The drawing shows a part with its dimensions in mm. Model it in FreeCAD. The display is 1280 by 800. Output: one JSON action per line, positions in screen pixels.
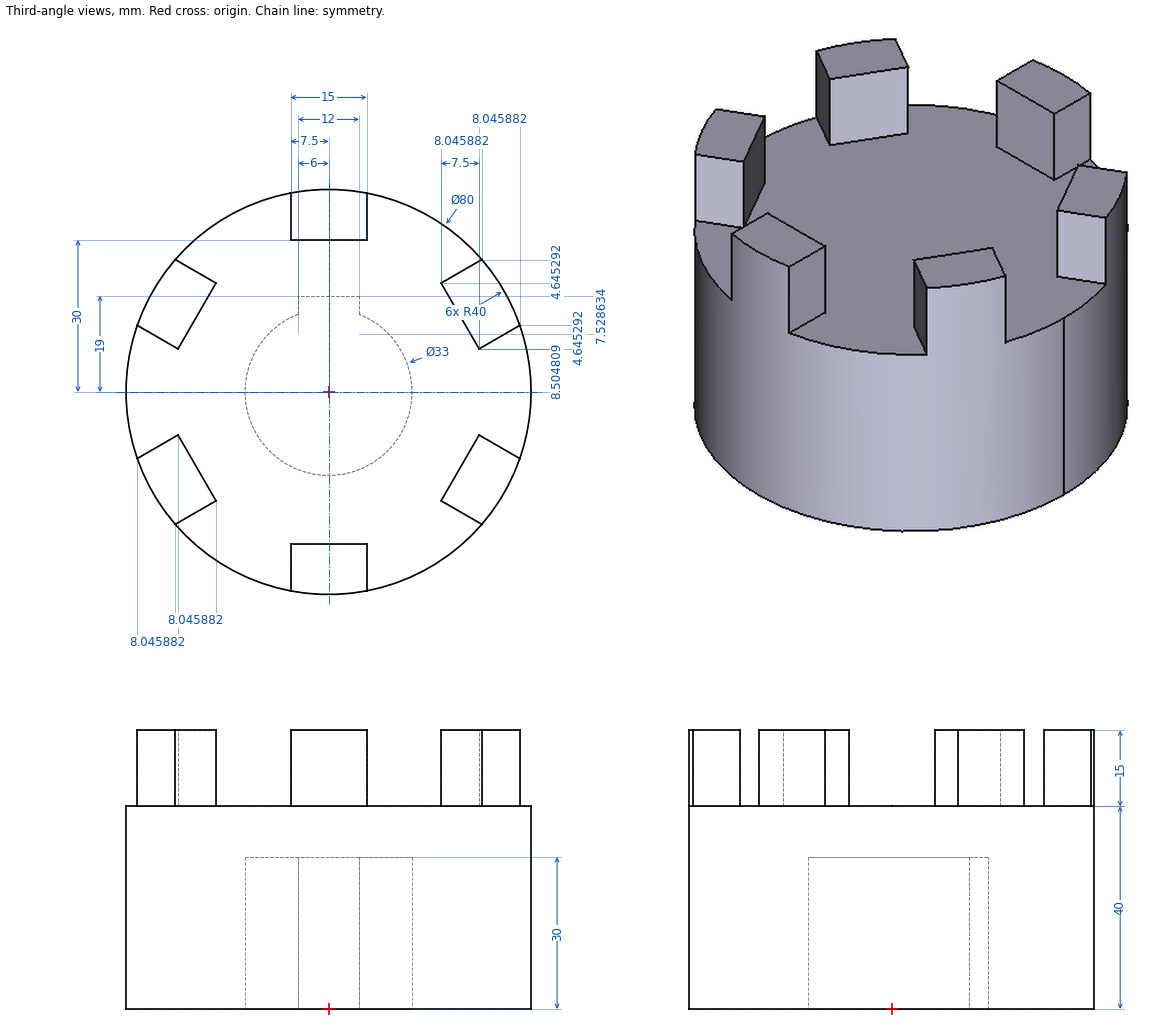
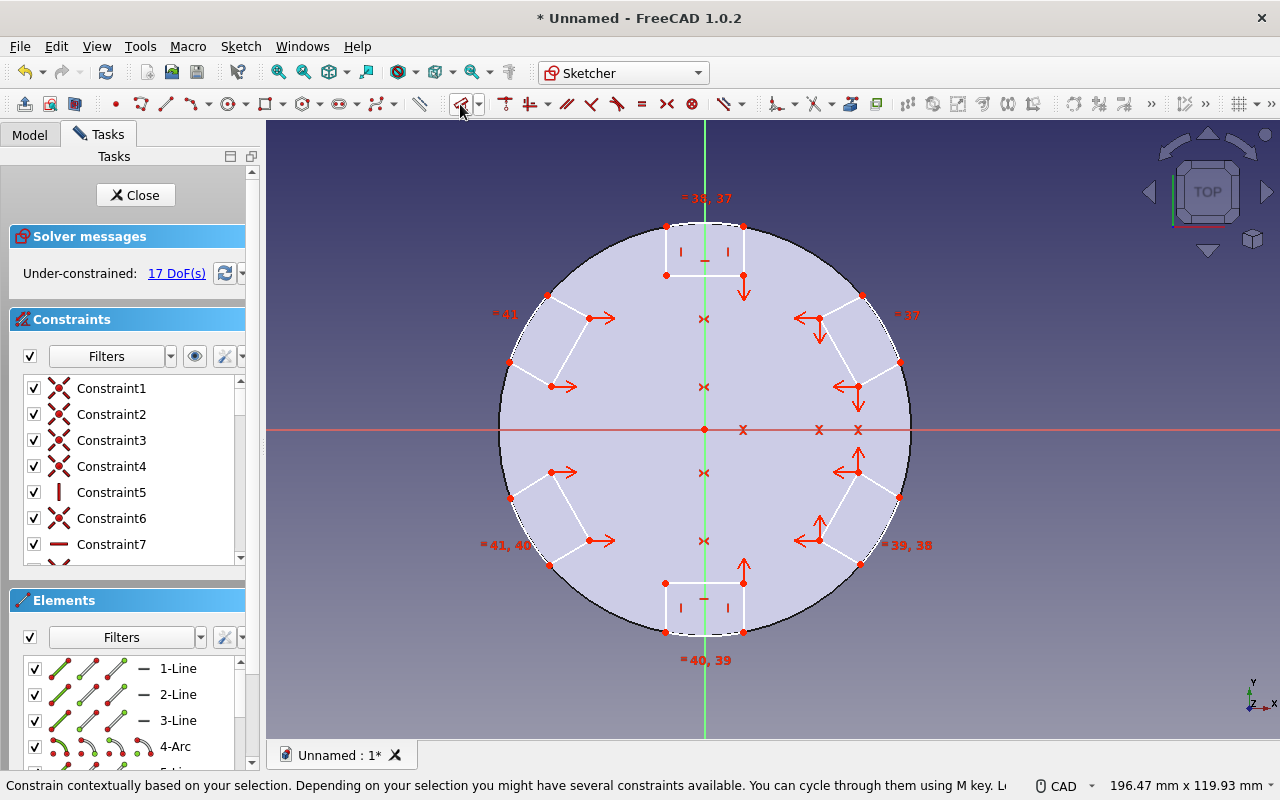
{"action": "left_click", "coordinate": [892, 341]}
{"action": "left_click", "coordinate": [921, 327]}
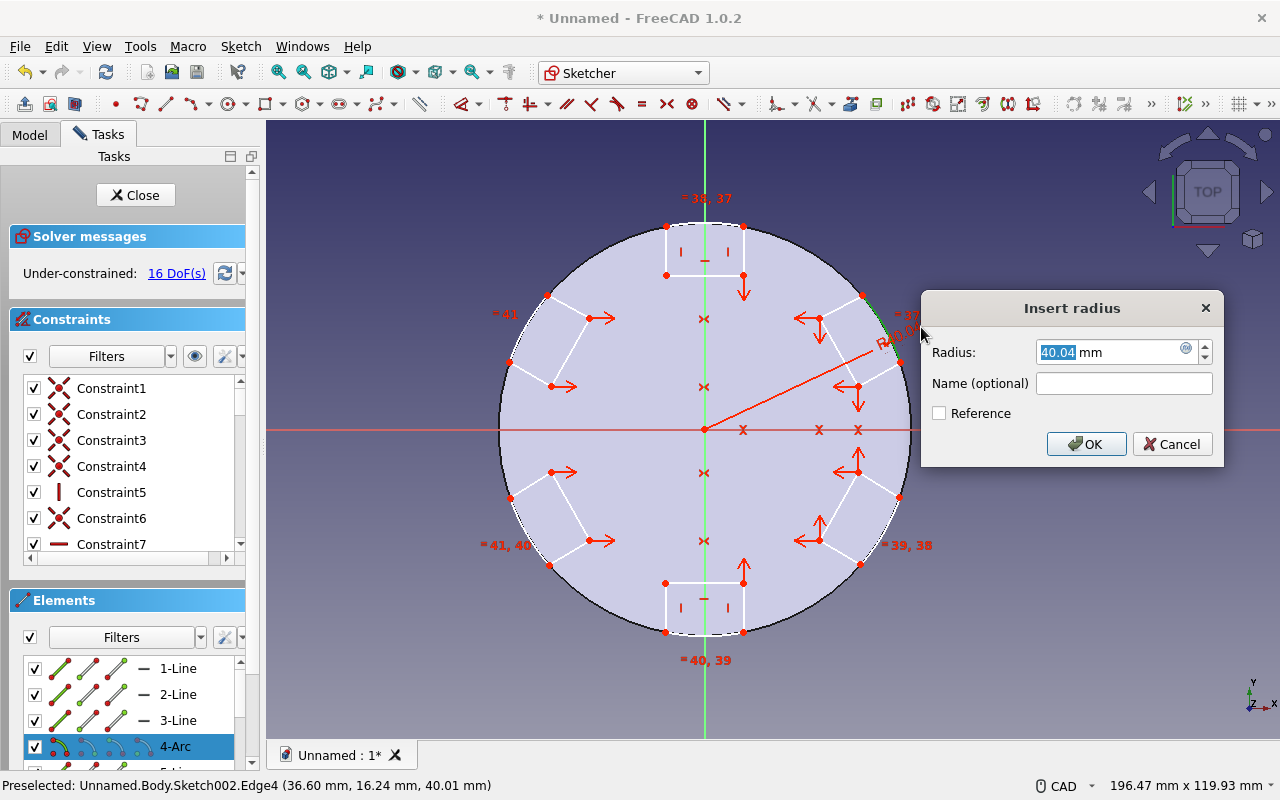
{"action": "type", "text": "40"}
{"action": "key", "text": "Return"}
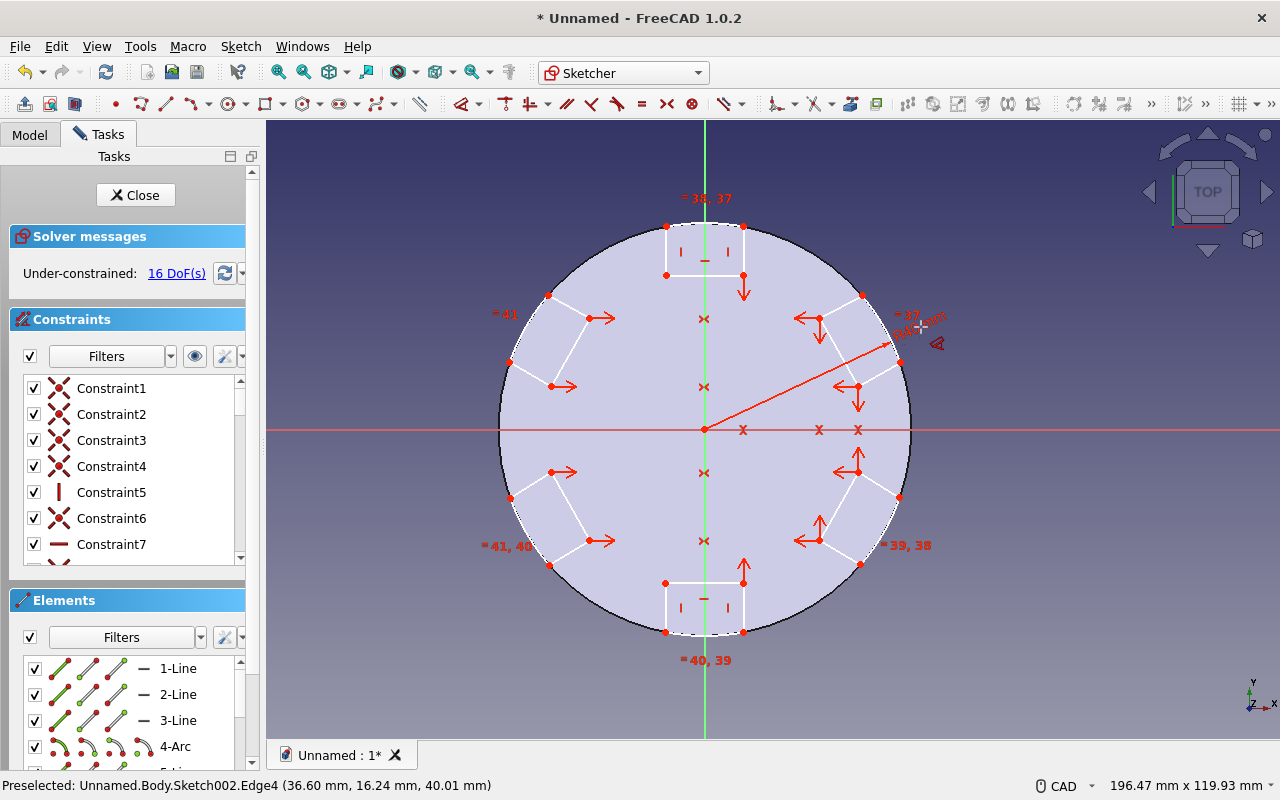
{"action": "left_click", "coordinate": [689, 276]}
{"action": "left_click", "coordinate": [687, 242]}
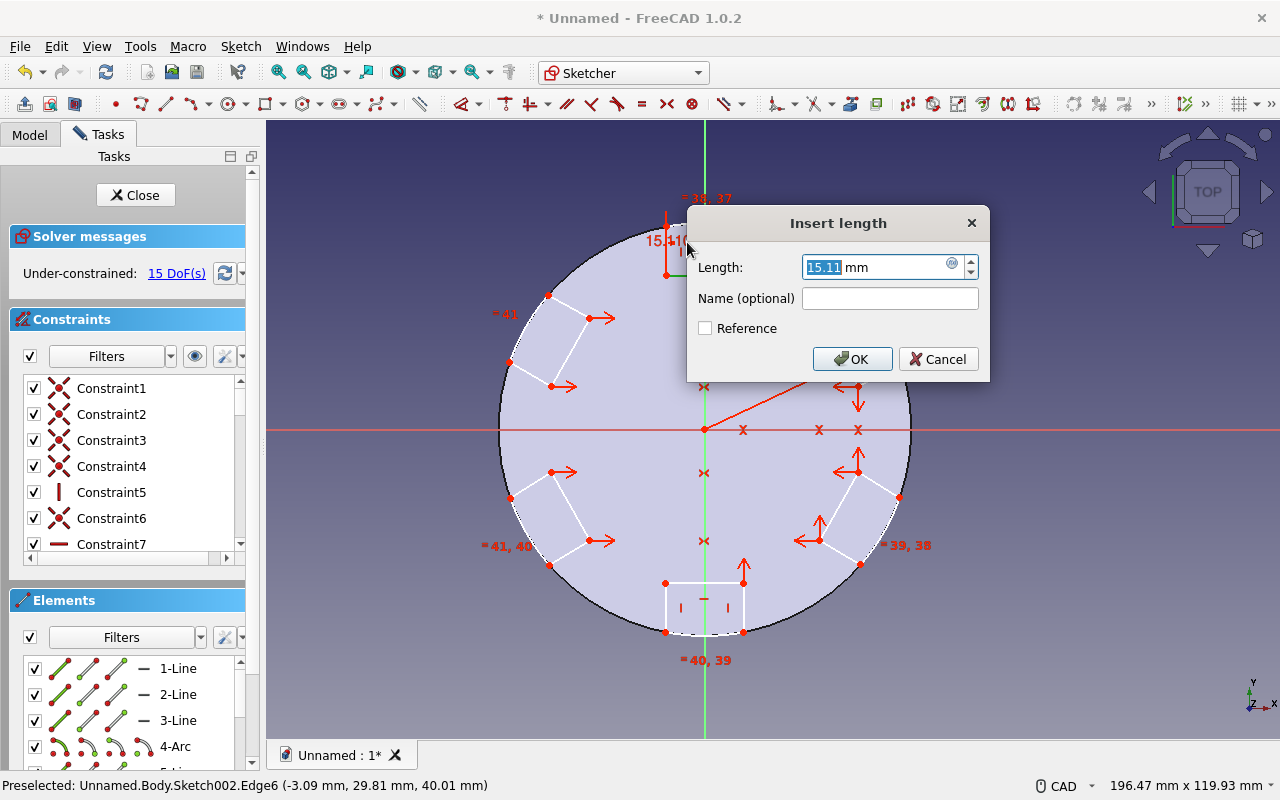
{"action": "type", "text": "15"}
{"action": "key", "text": "Return"}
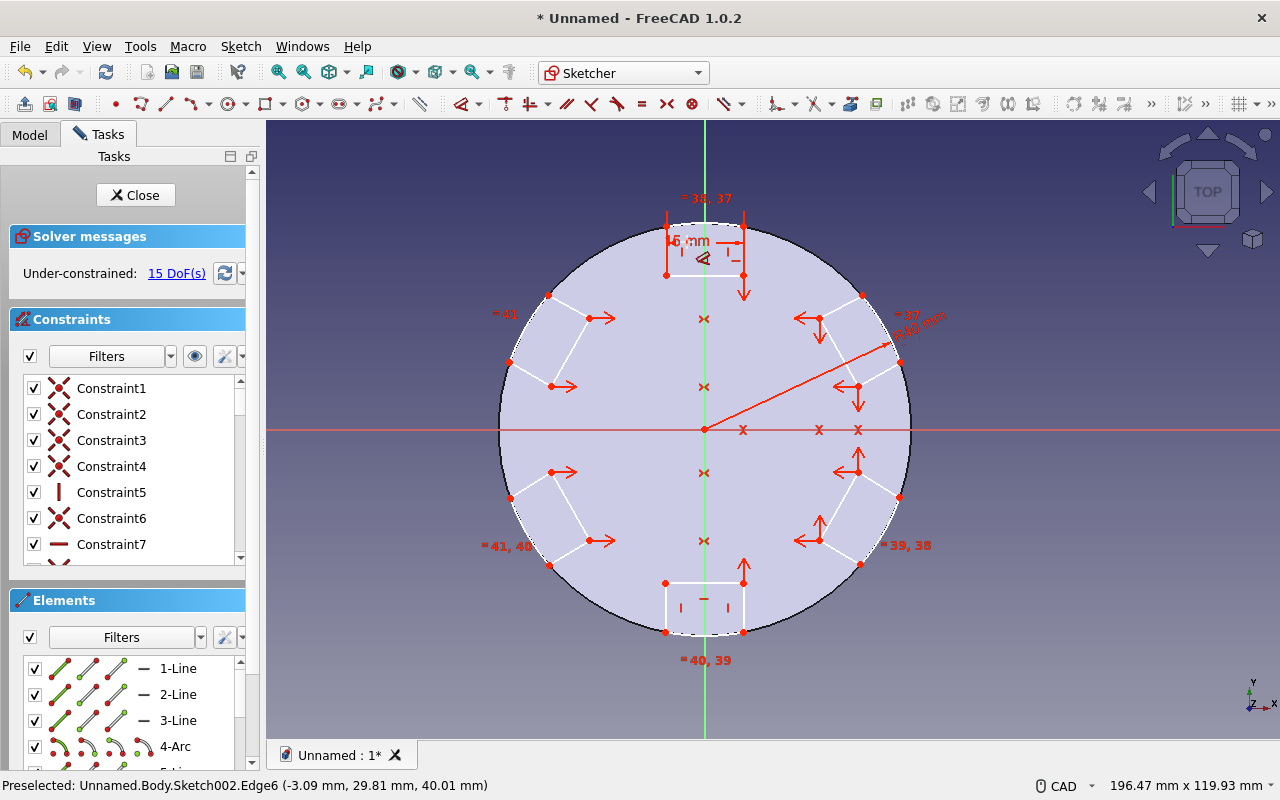
{"action": "left_click", "coordinate": [721, 583]}
{"action": "left_click", "coordinate": [687, 617]}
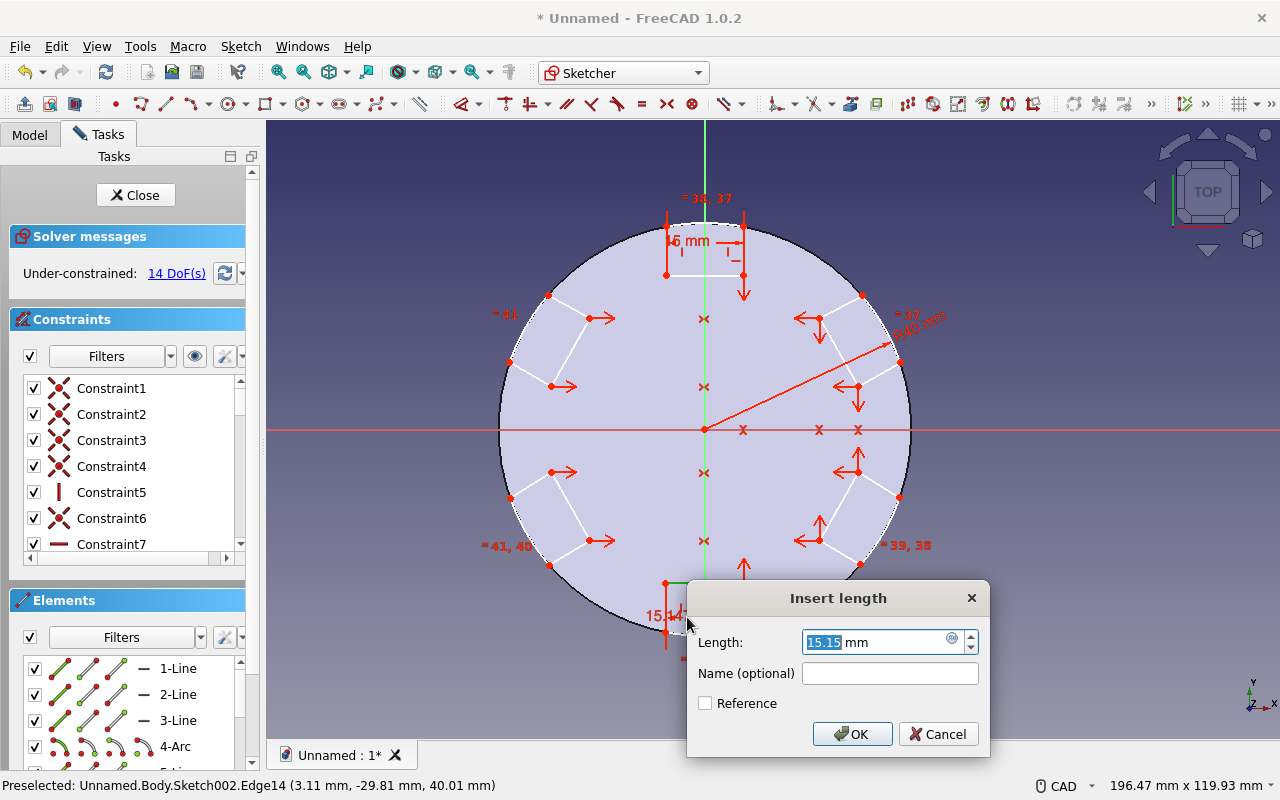
{"action": "type", "text": "15"}
{"action": "key", "text": "Return"}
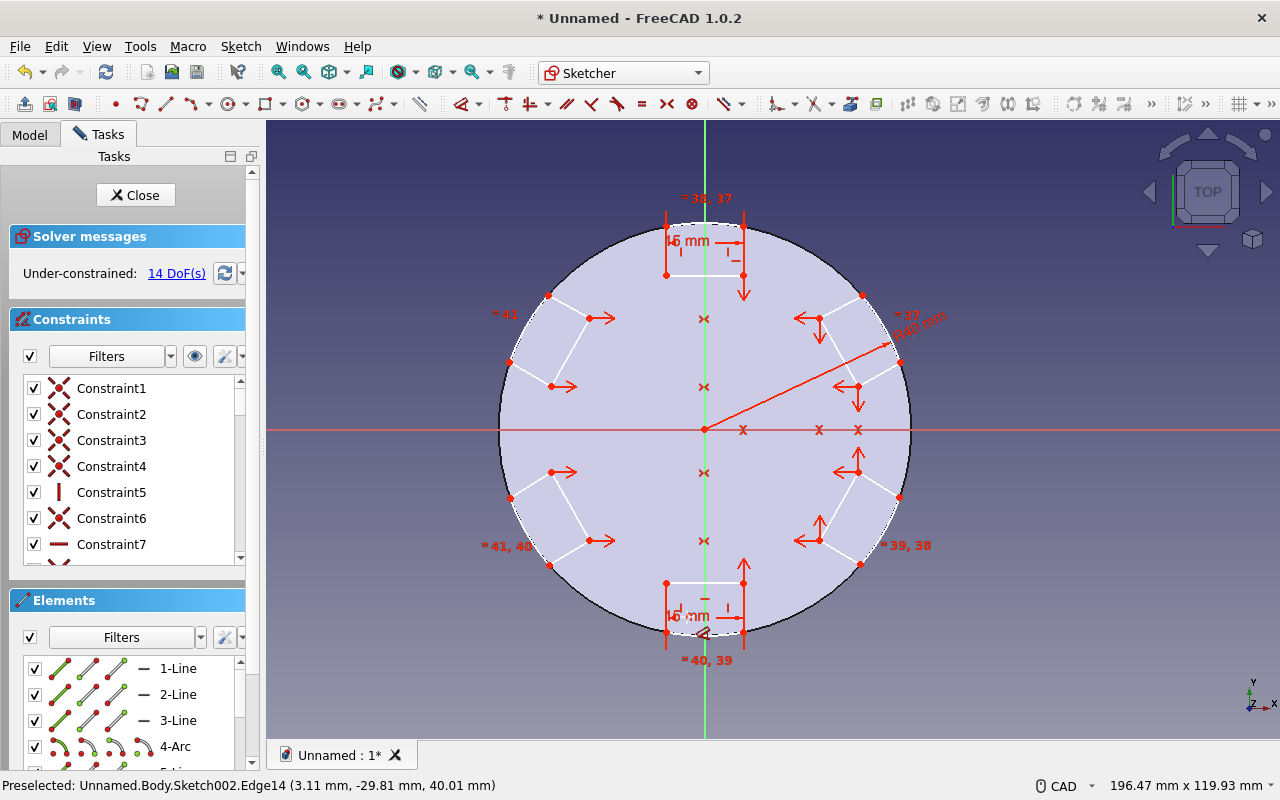
{"action": "left_click", "coordinate": [666, 276]}
{"action": "left_click", "coordinate": [632, 353]}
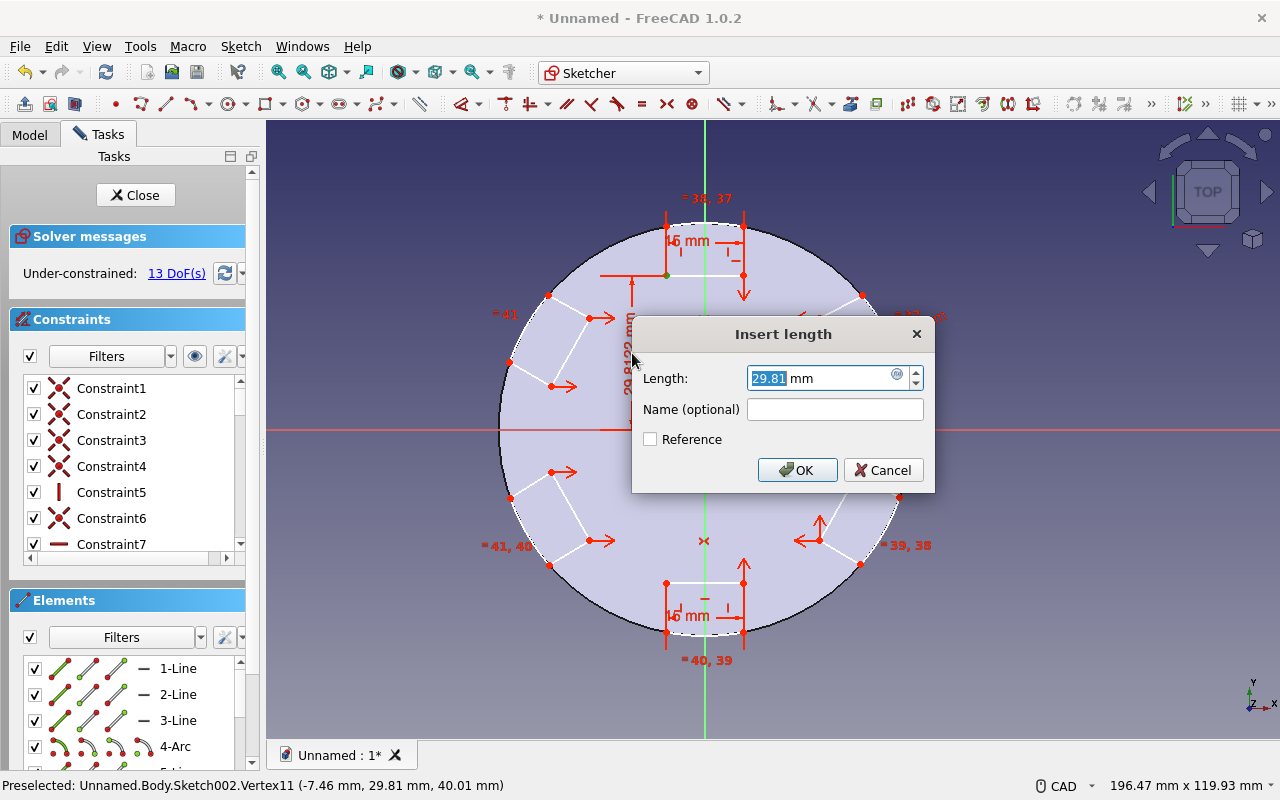
{"action": "type", "text": "30"}
{"action": "key", "text": "Return"}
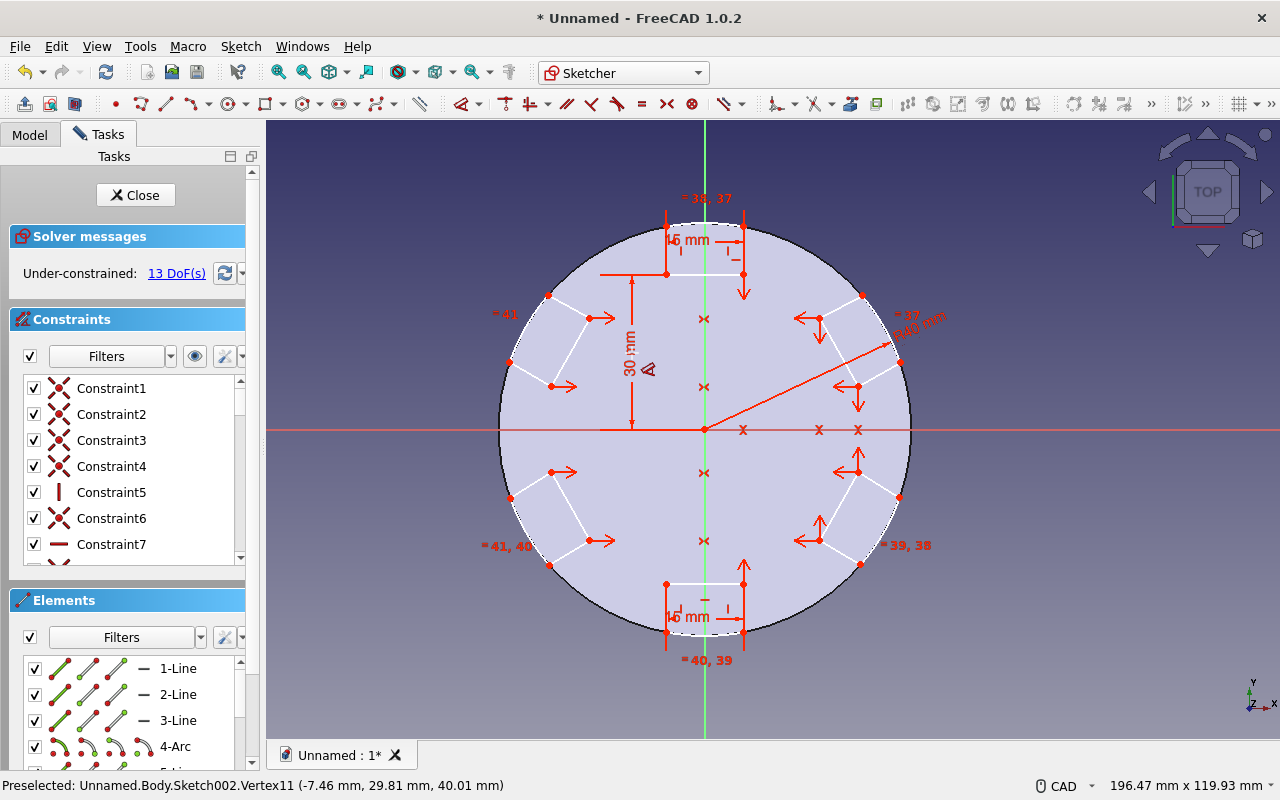
{"action": "left_click", "coordinate": [666, 227]}
{"action": "left_click", "coordinate": [686, 193]}